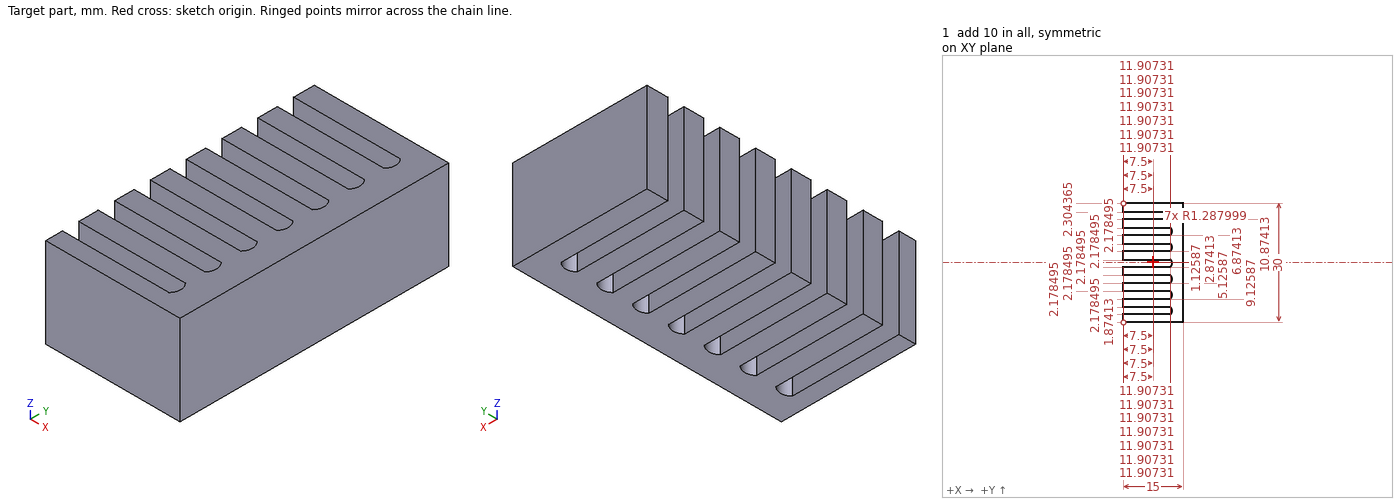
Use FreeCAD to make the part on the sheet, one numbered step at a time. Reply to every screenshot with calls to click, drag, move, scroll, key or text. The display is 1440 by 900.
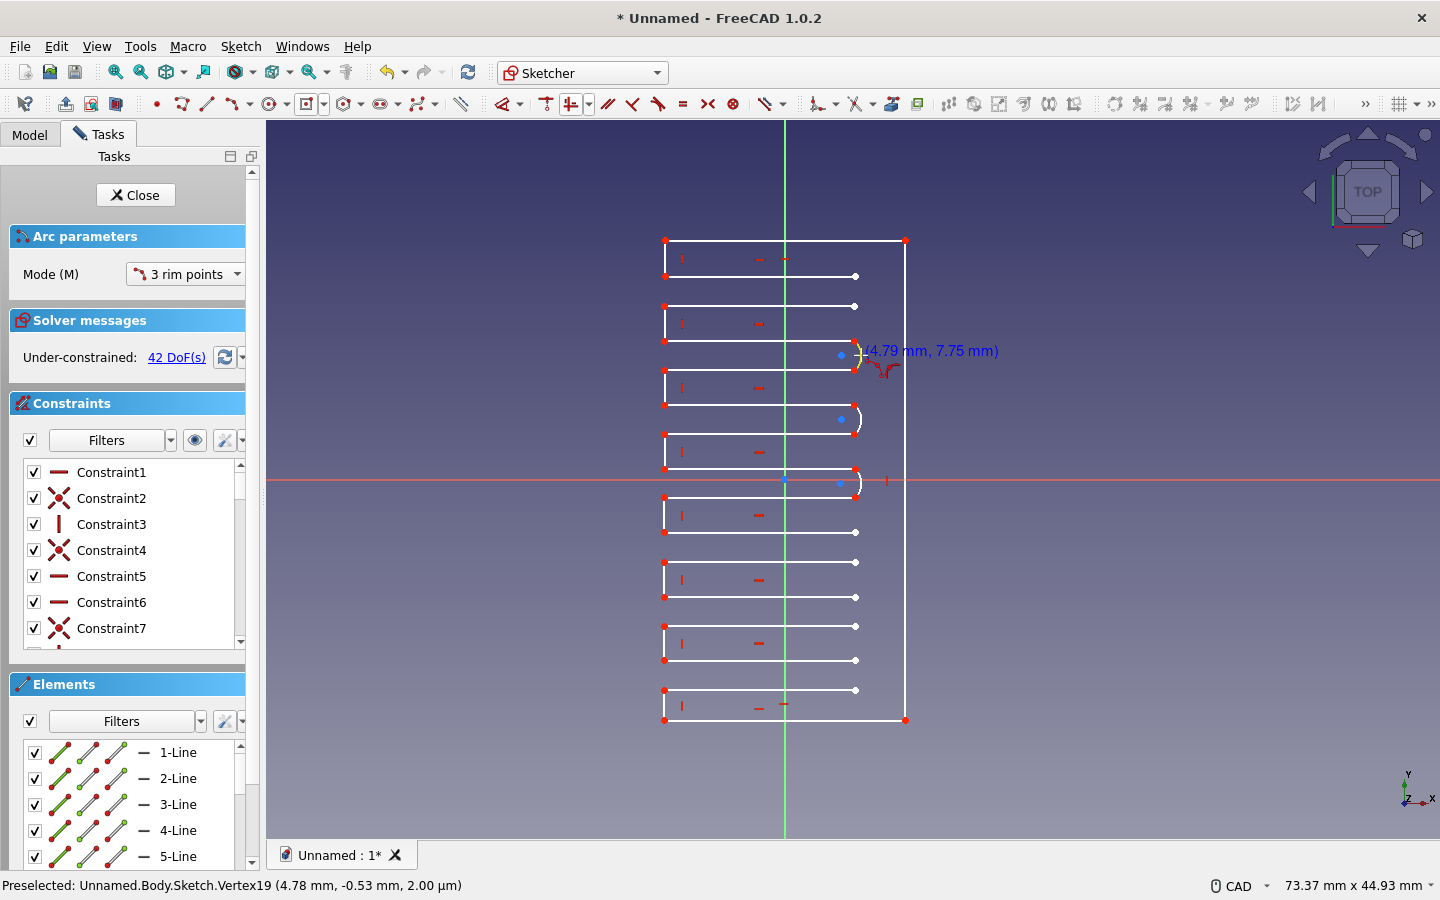
click(855, 533)
click(855, 562)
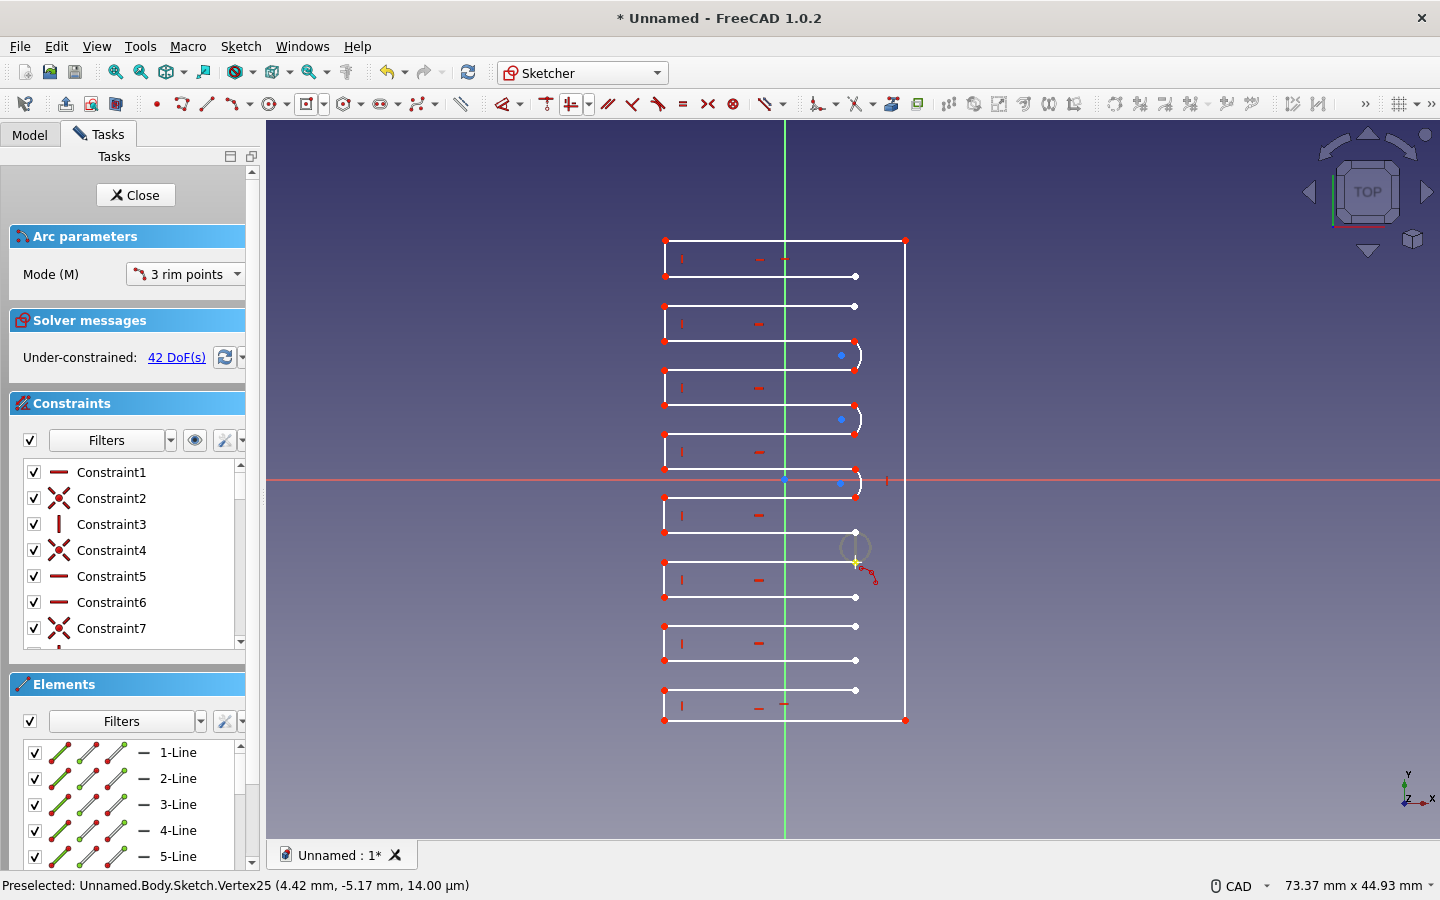
scroll(861, 547, up, 5)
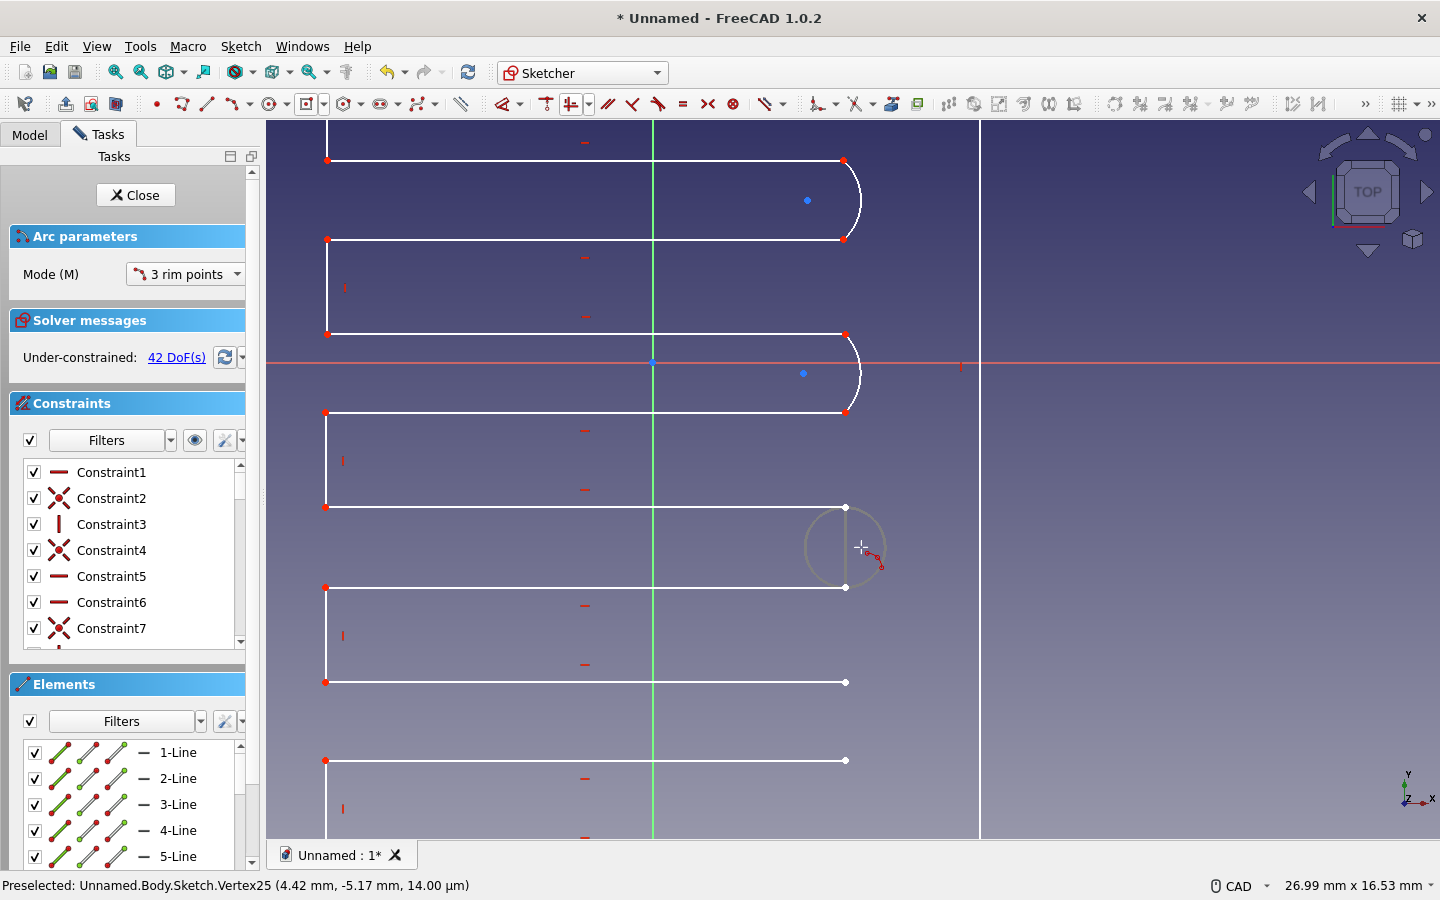
click(861, 546)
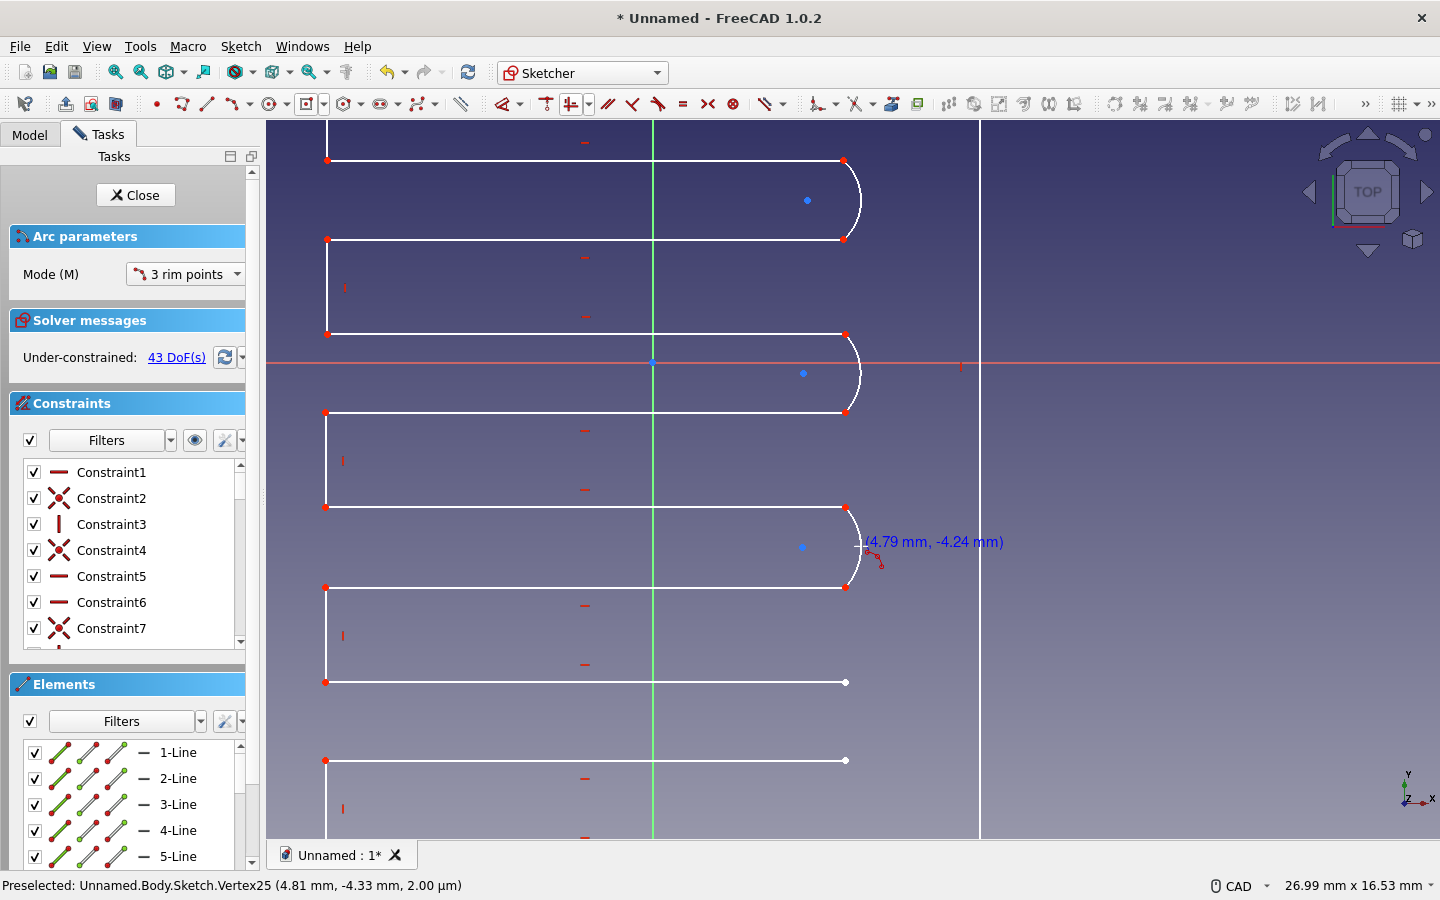
click(845, 682)
click(845, 761)
click(861, 720)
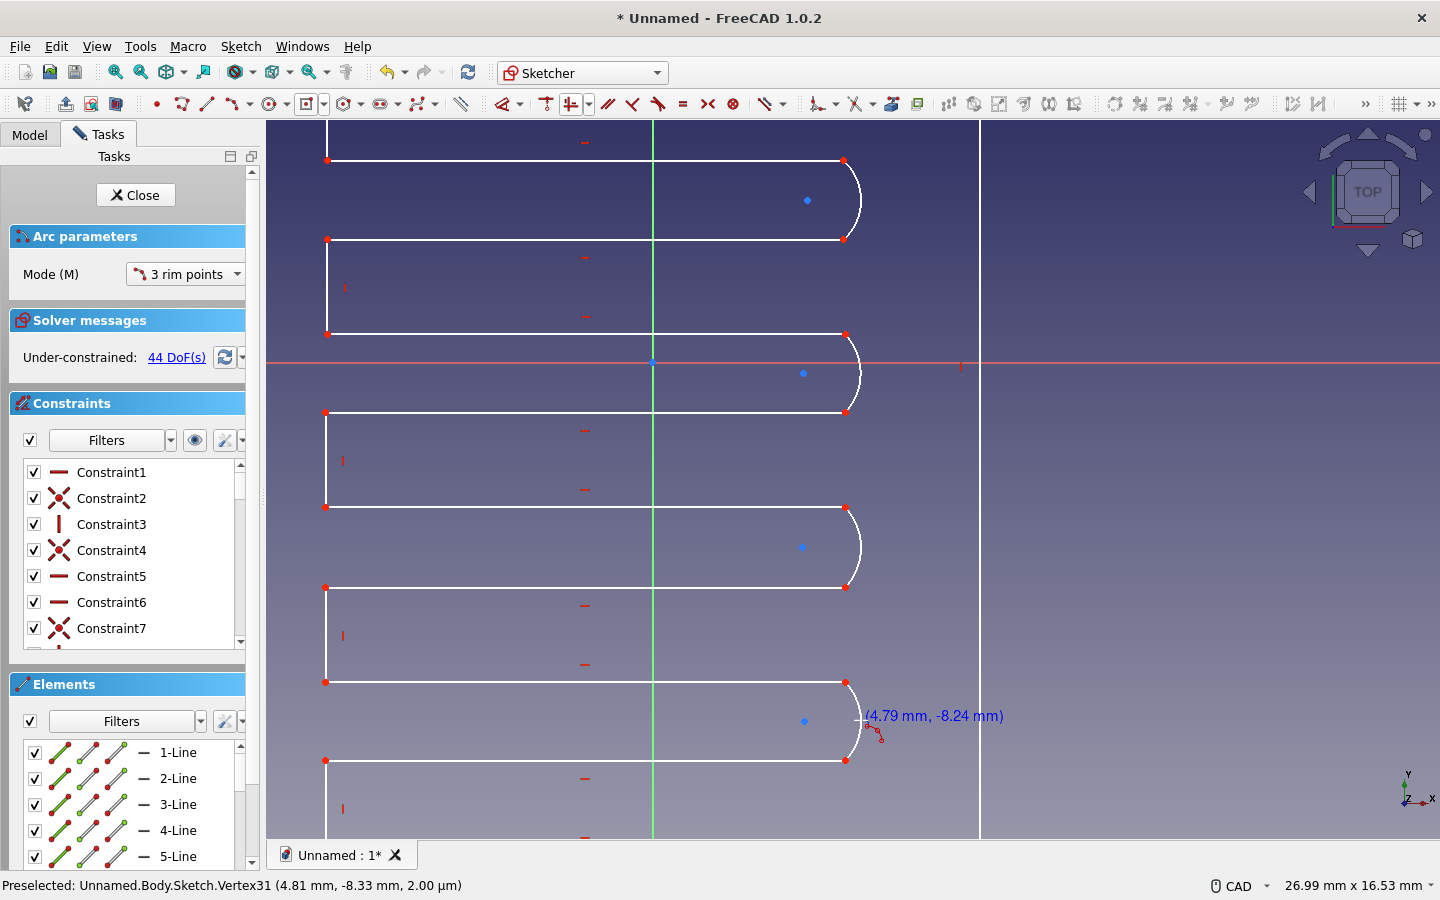
scroll(861, 547, down, 5)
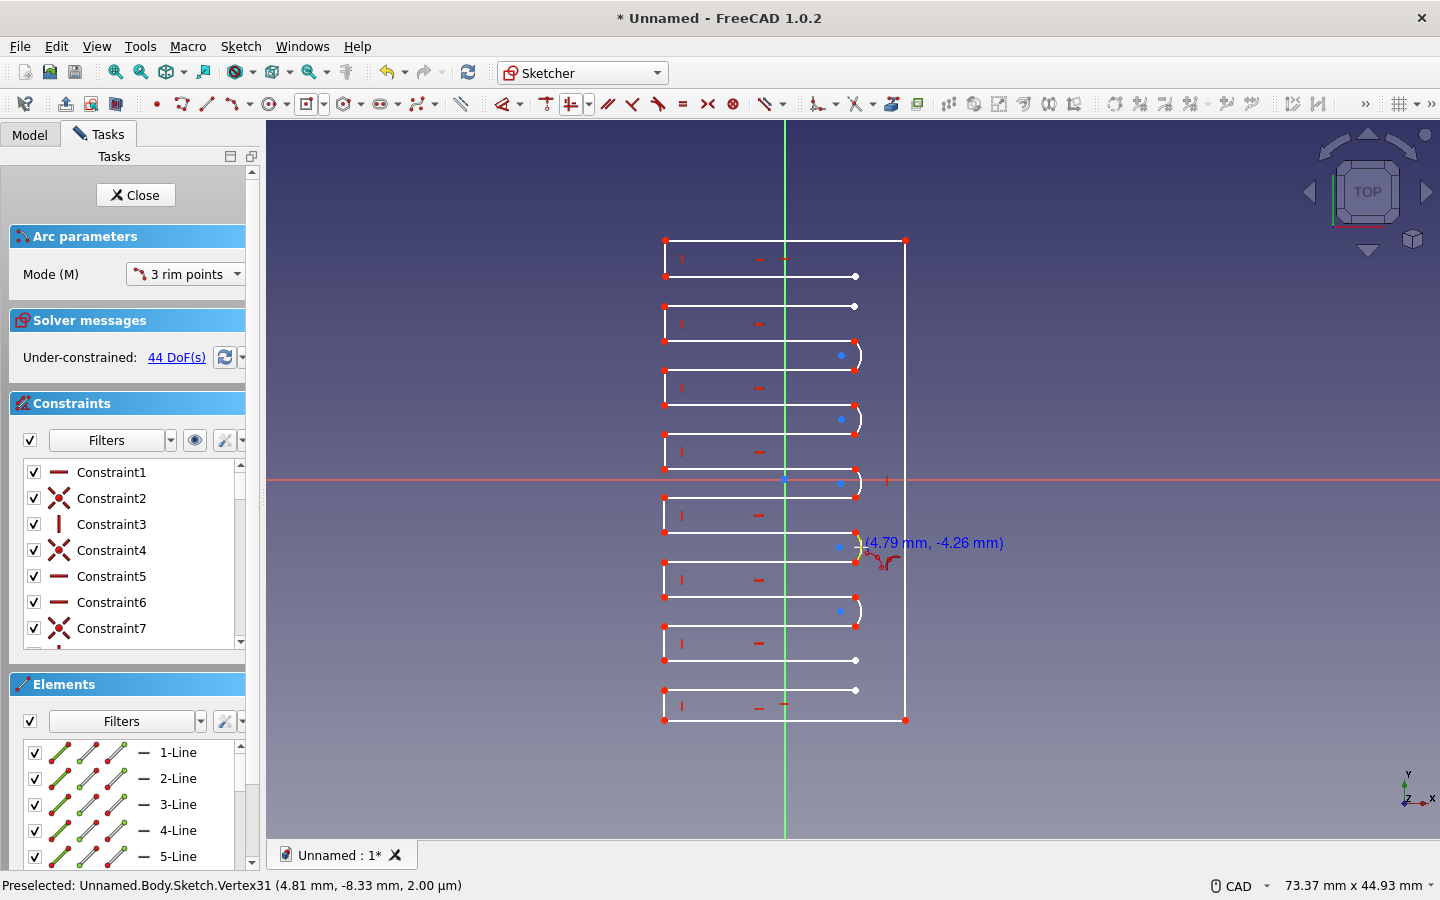
click(855, 661)
click(855, 690)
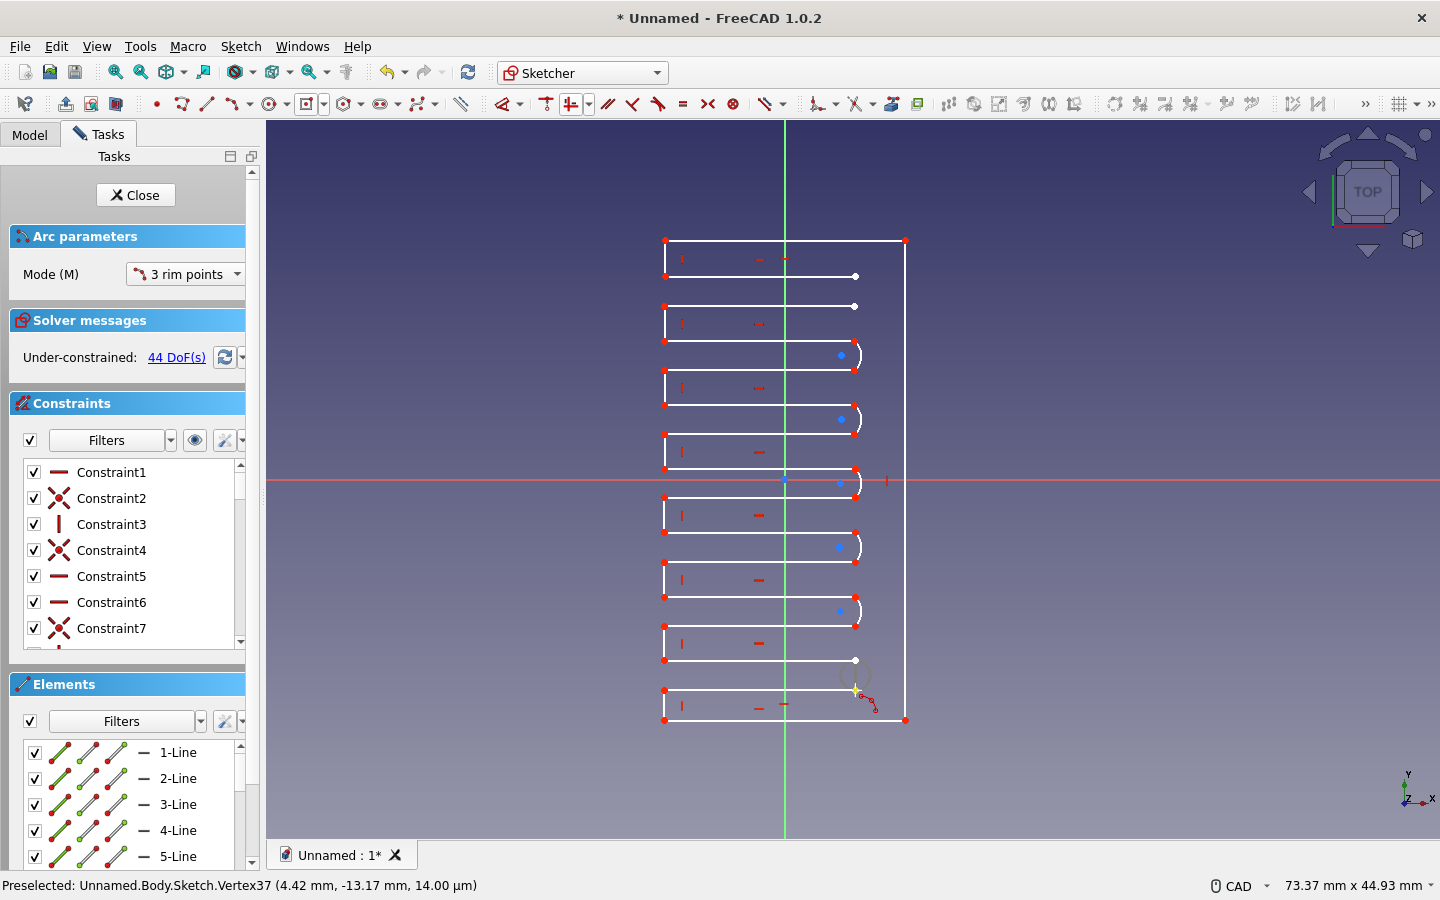
scroll(861, 675, up, 5)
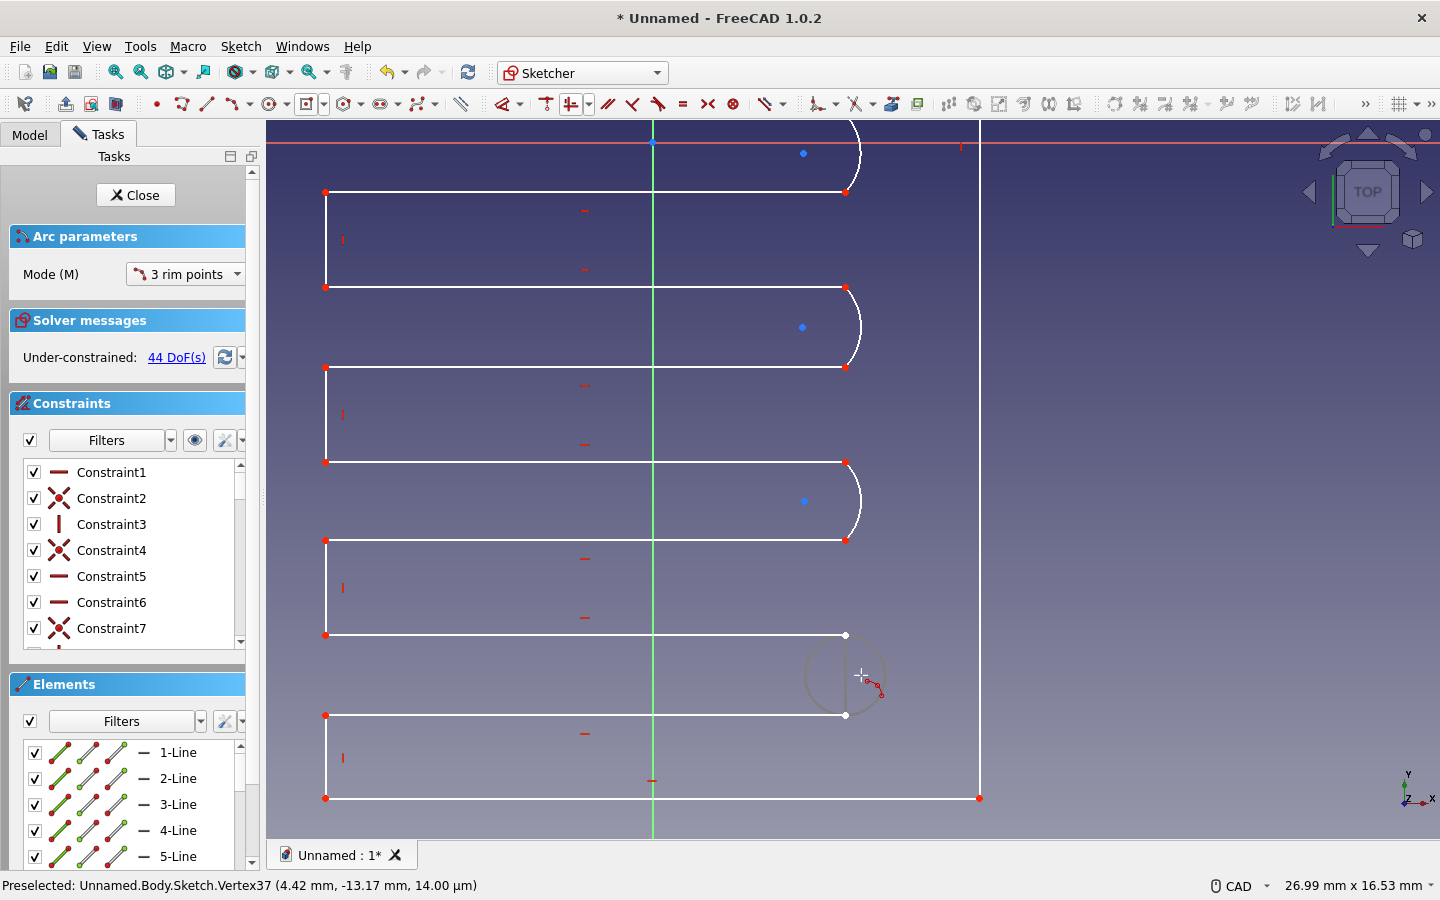
click(861, 674)